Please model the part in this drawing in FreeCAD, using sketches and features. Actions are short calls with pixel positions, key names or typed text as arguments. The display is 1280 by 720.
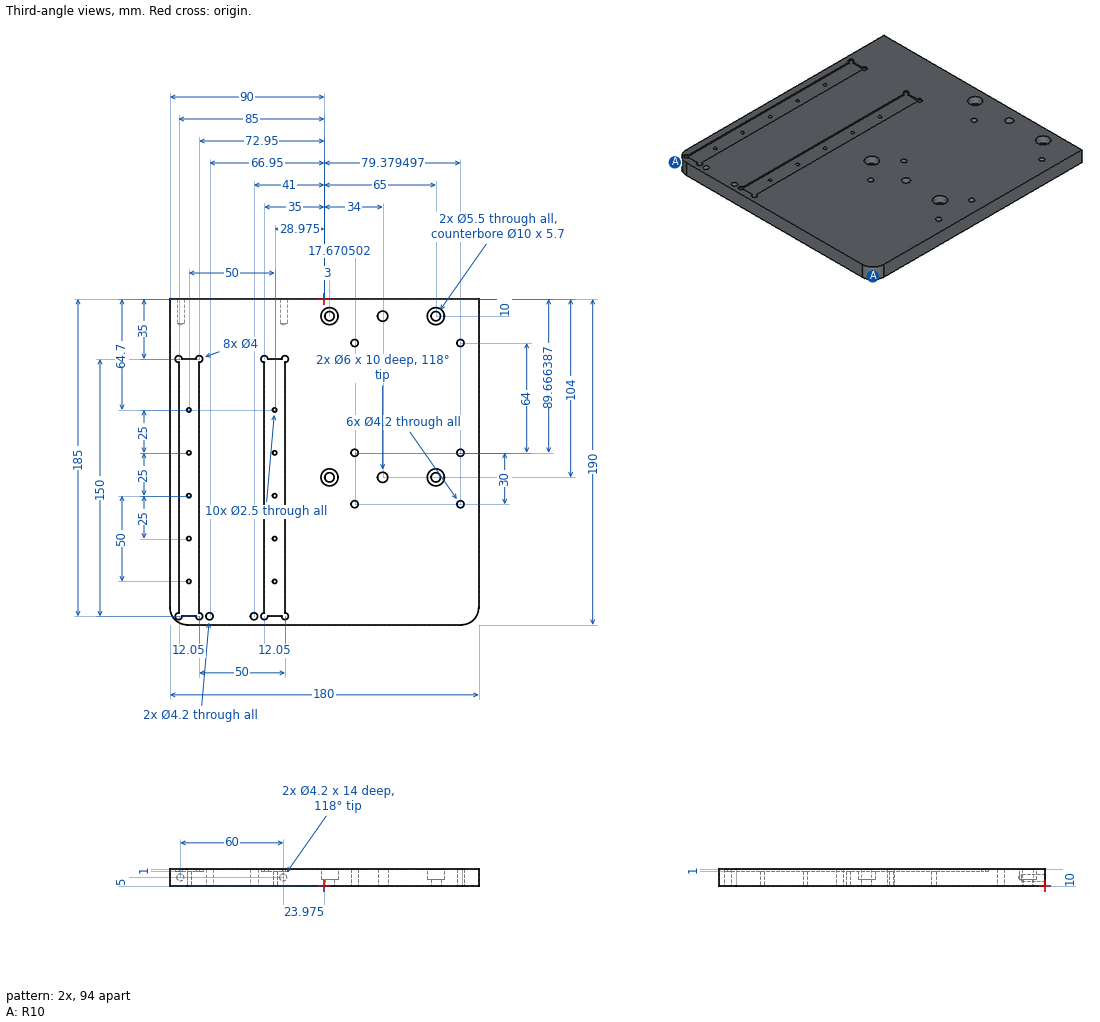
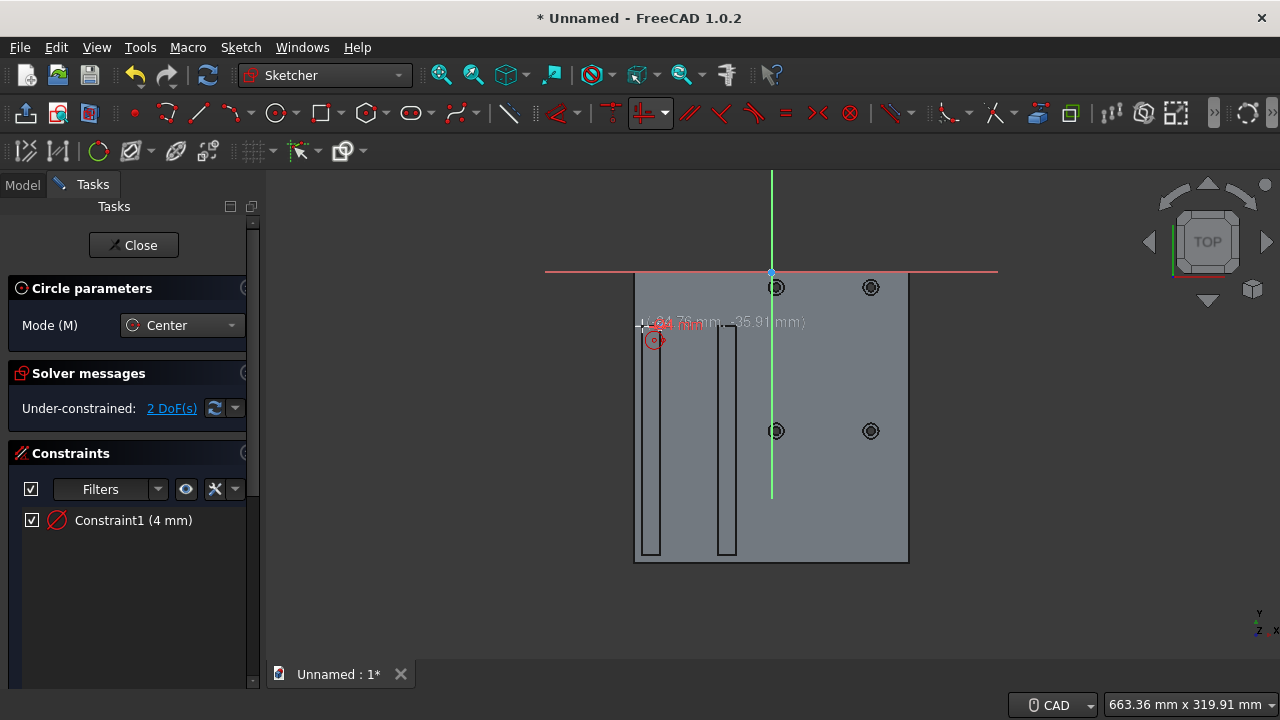
click(642, 326)
move(639, 323)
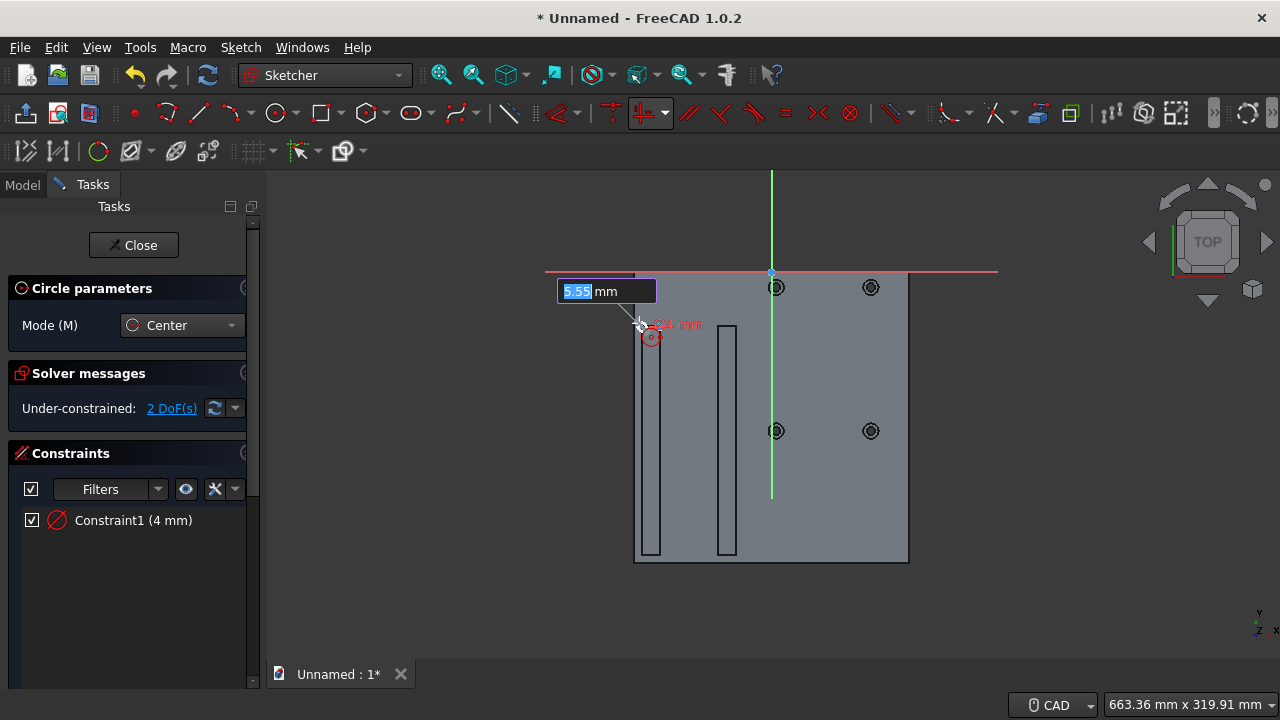
text(4)
key(Return)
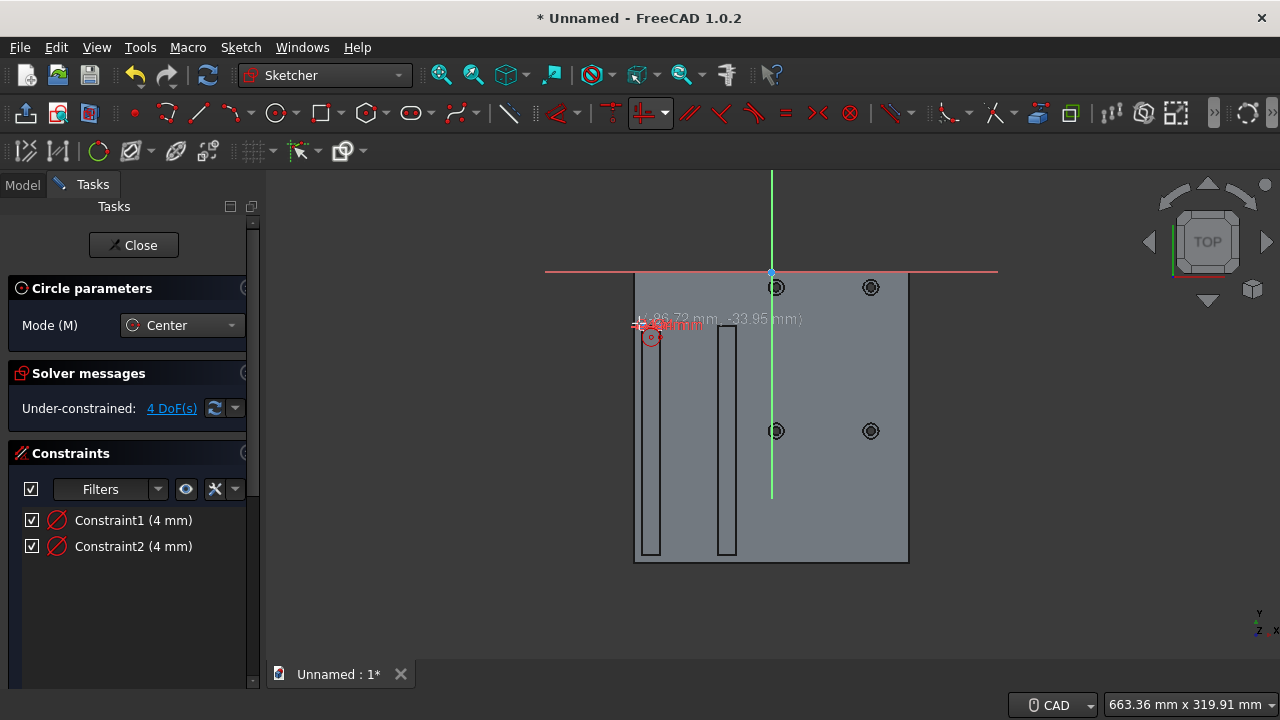
scroll(642, 555, up, 11)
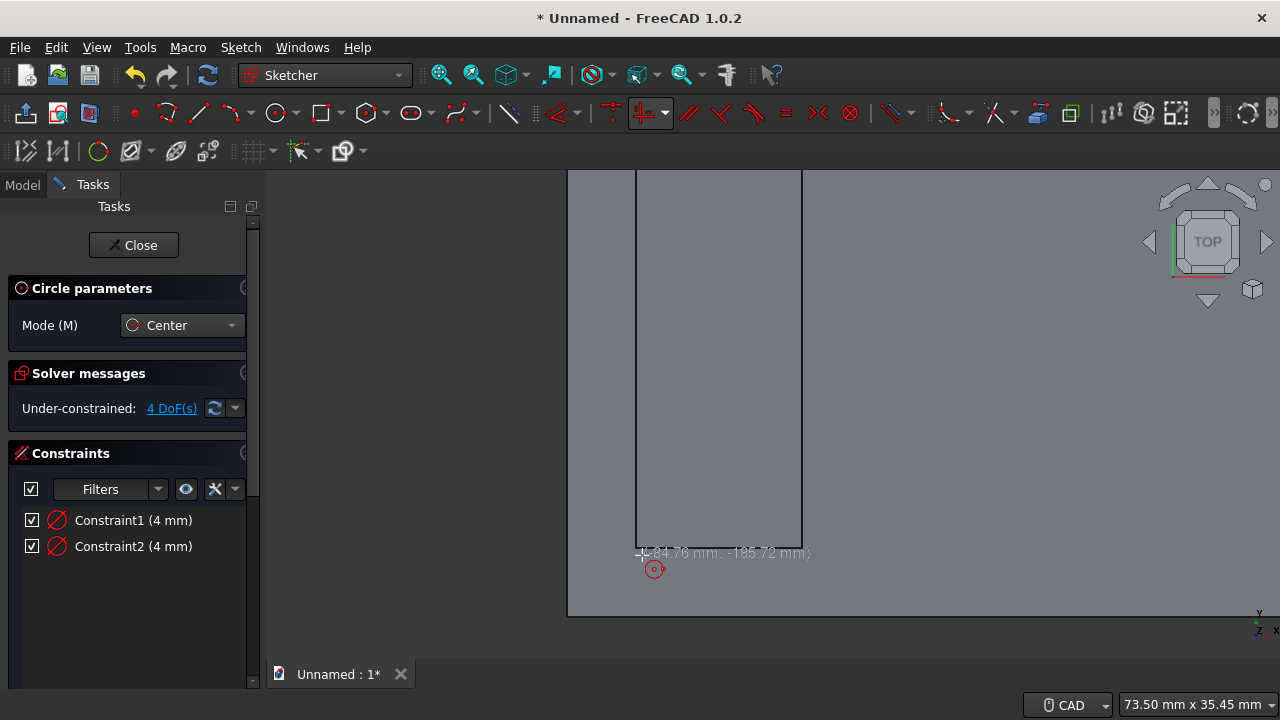
scroll(642, 555, down, 11)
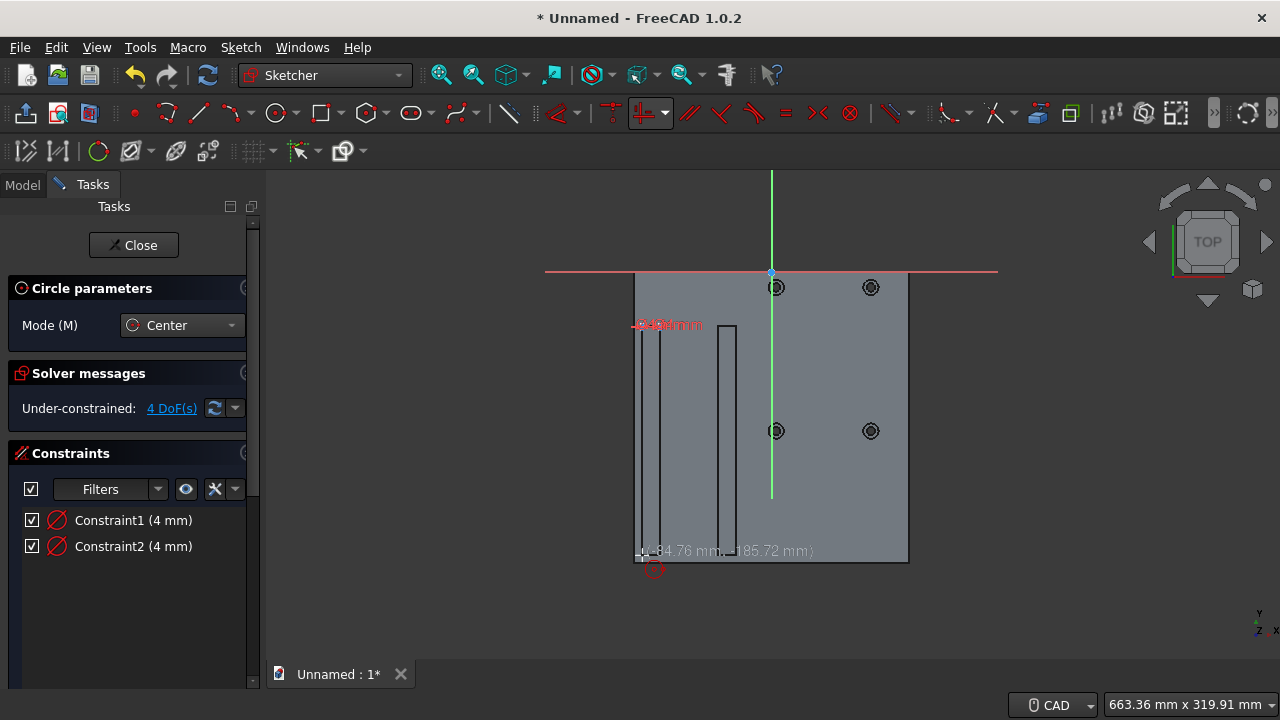
click(642, 555)
move(644, 553)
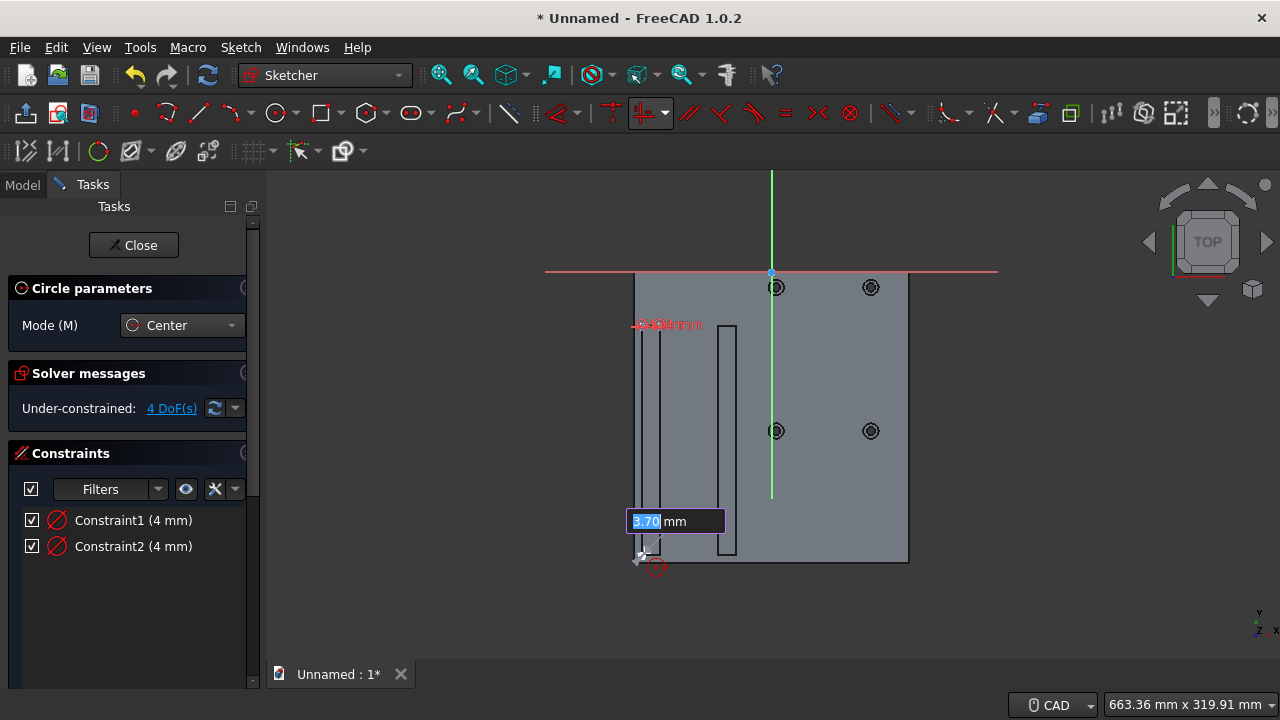
text(4)
key(Return)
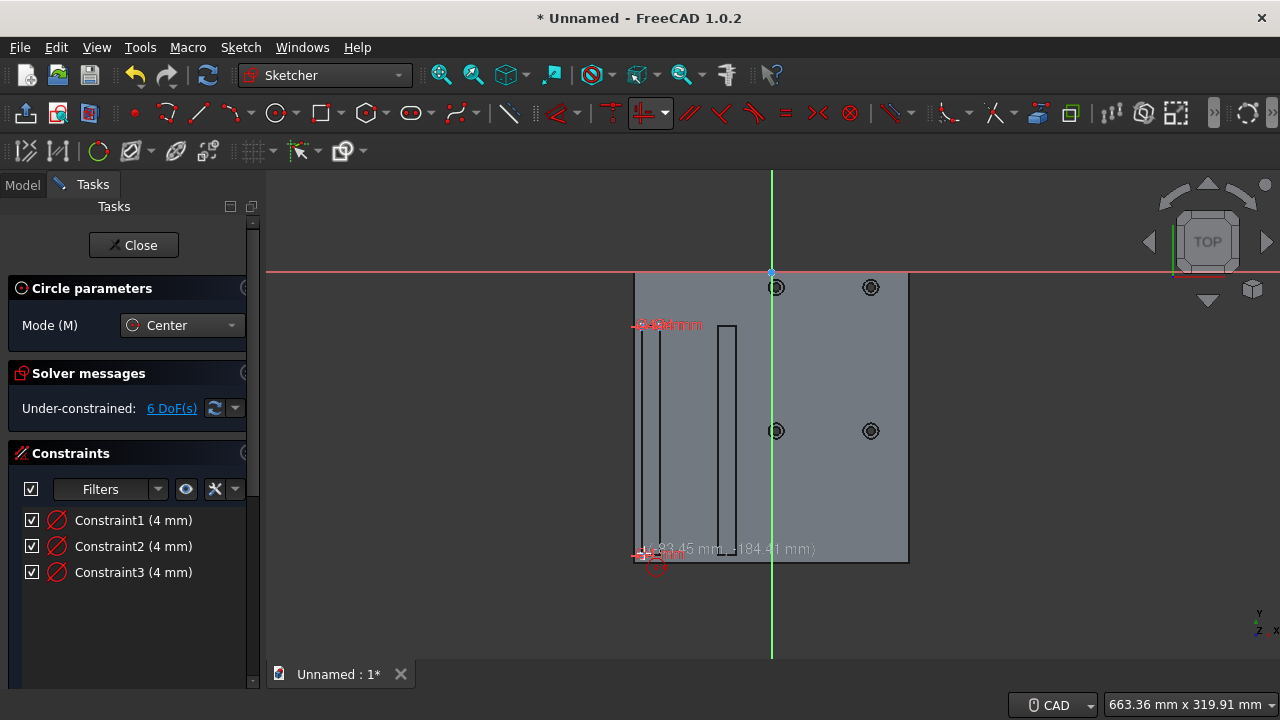
scroll(660, 555, up, 11)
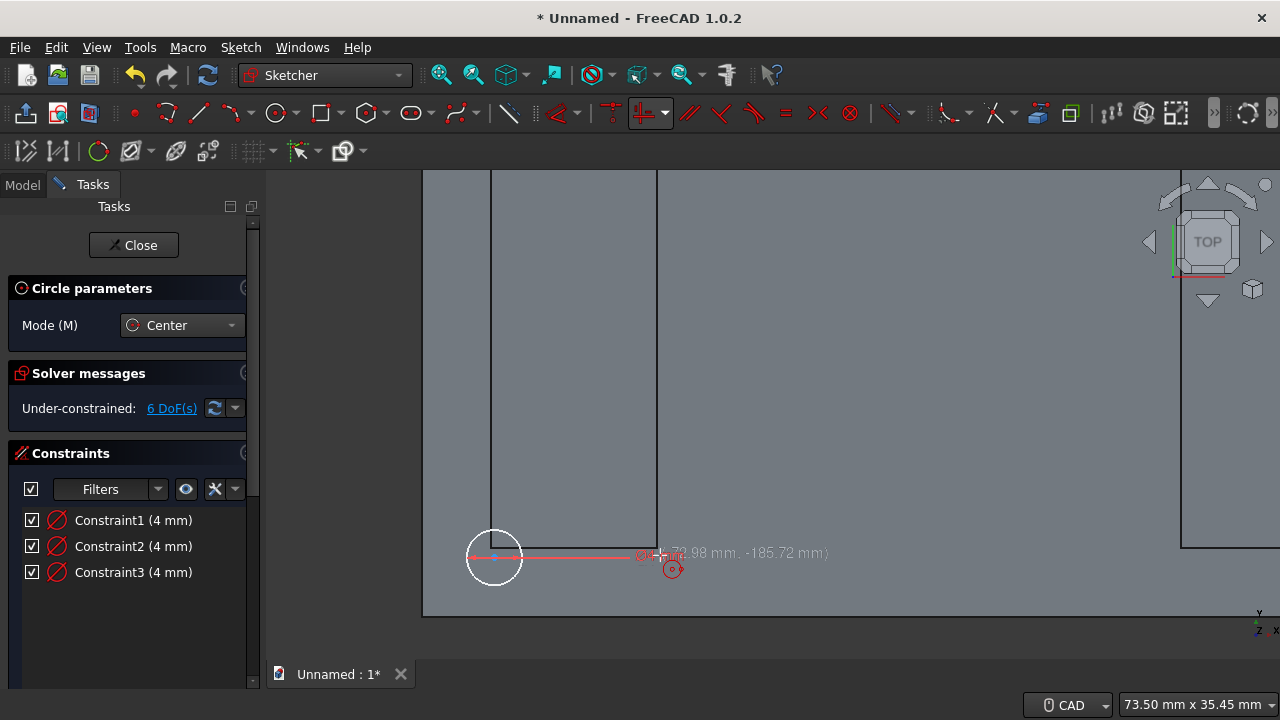
scroll(660, 555, down, 11)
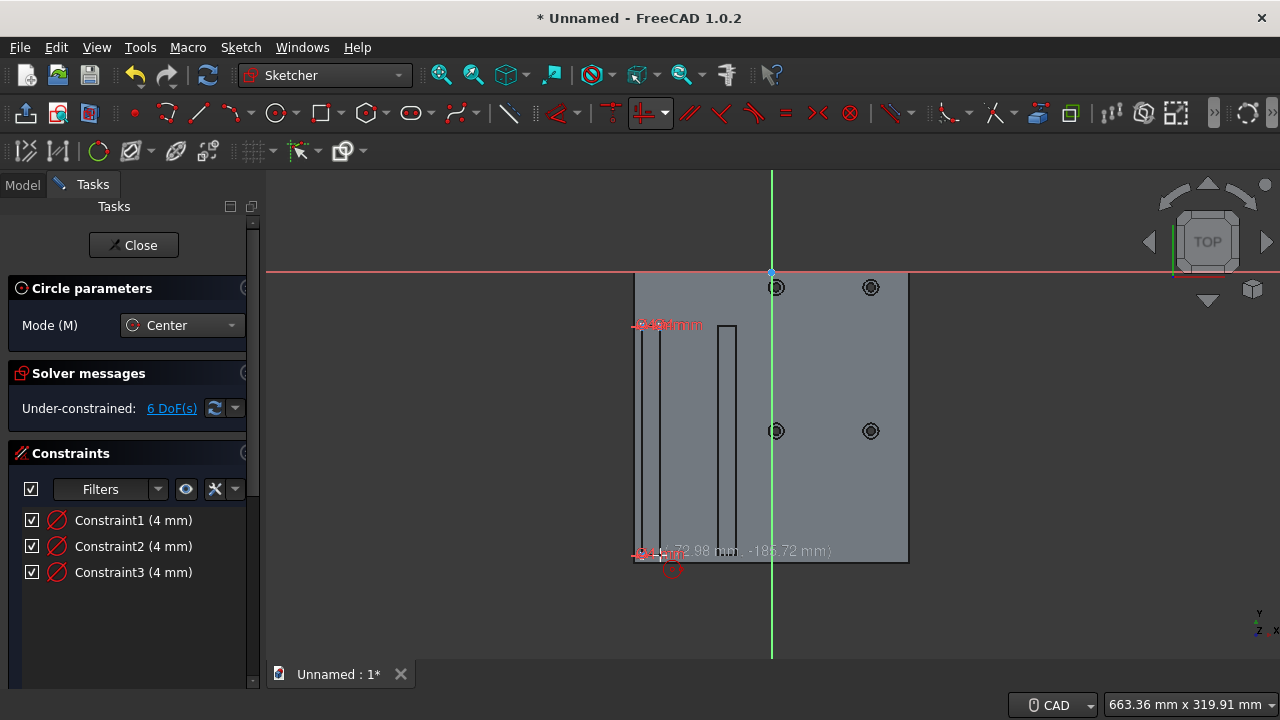
click(660, 555)
move(662, 553)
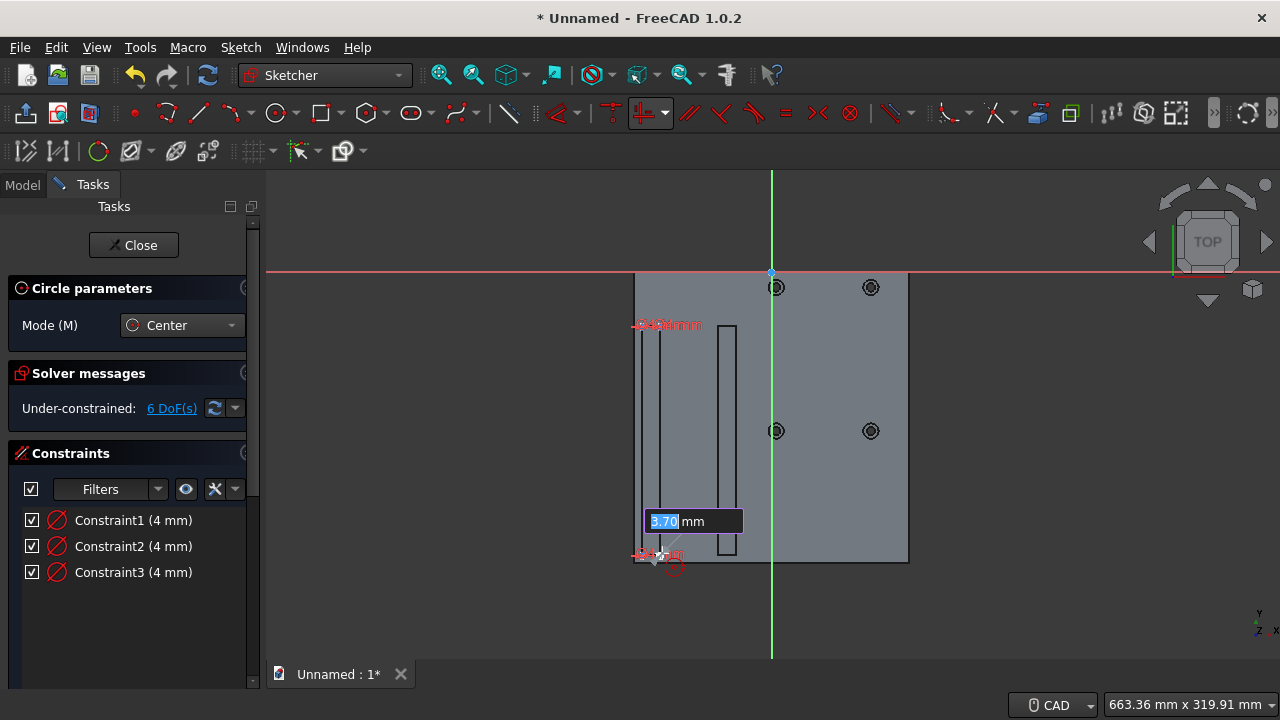
text(4)
key(Return)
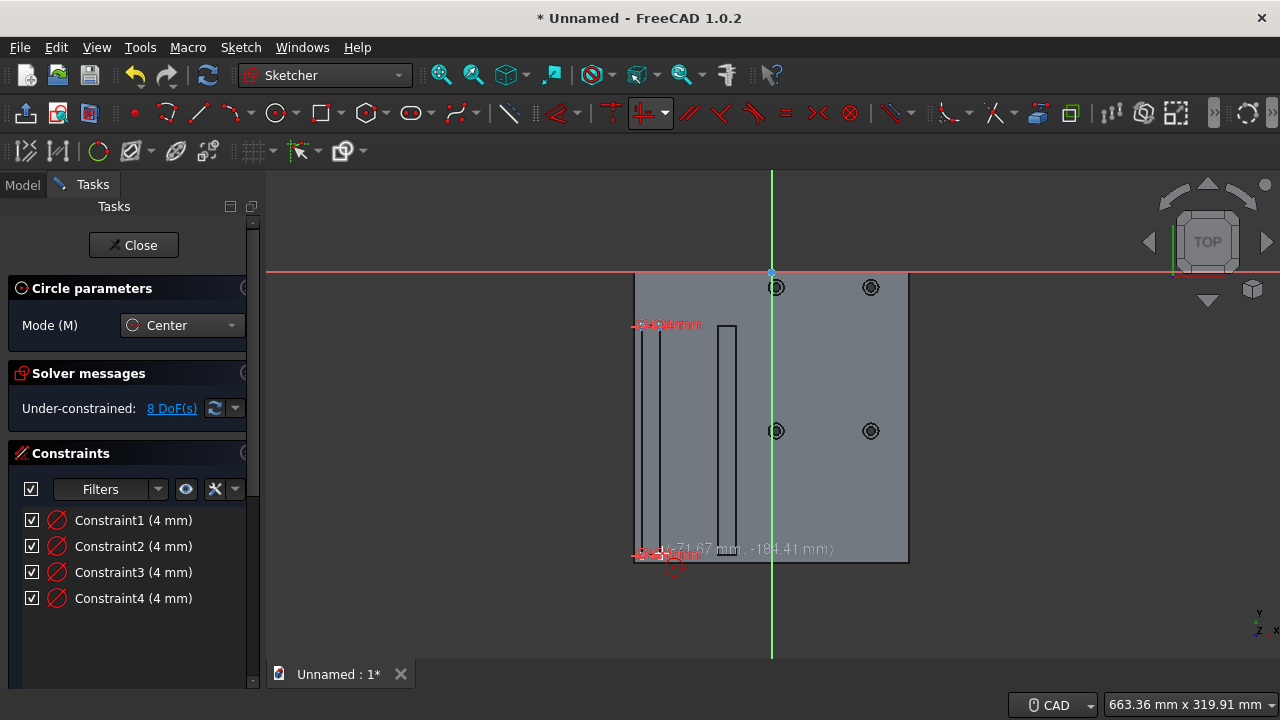
scroll(718, 555, up, 11)